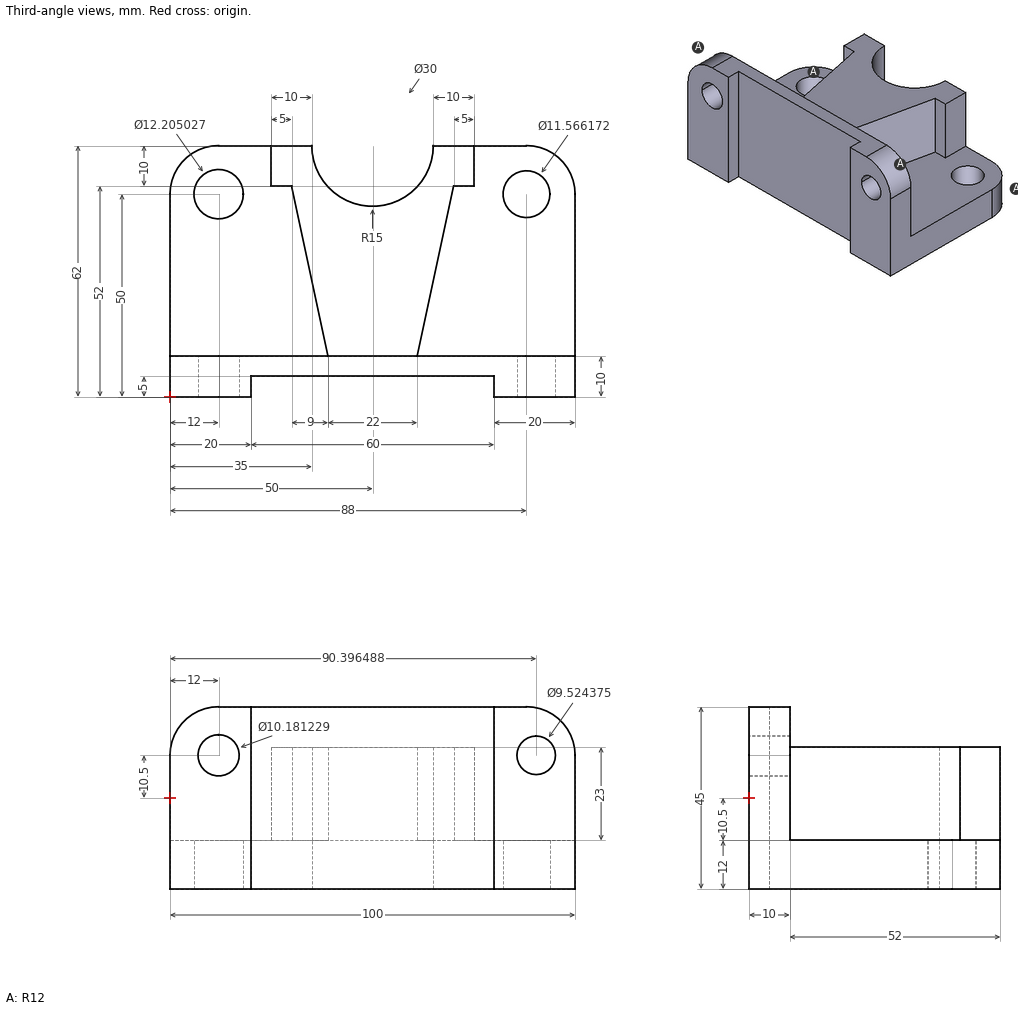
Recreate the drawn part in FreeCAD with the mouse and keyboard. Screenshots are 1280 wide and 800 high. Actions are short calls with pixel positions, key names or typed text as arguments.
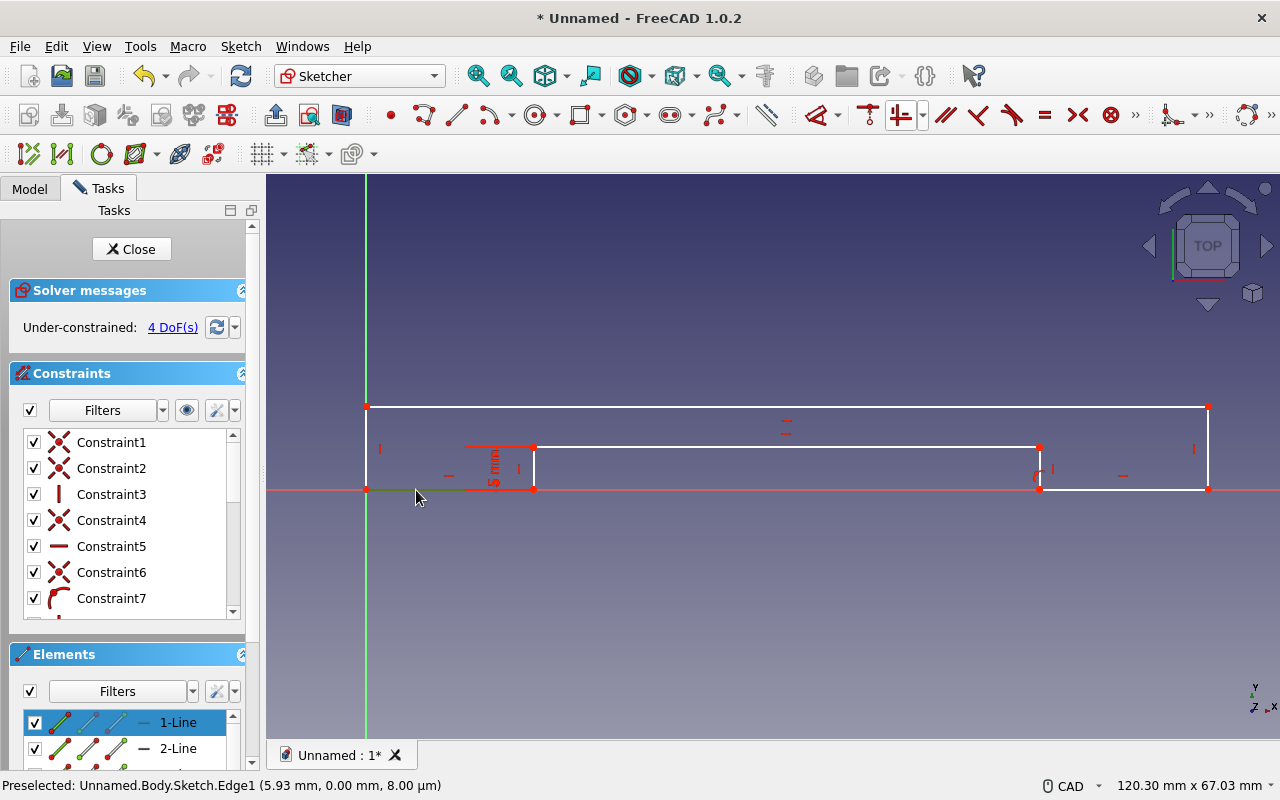
key(l)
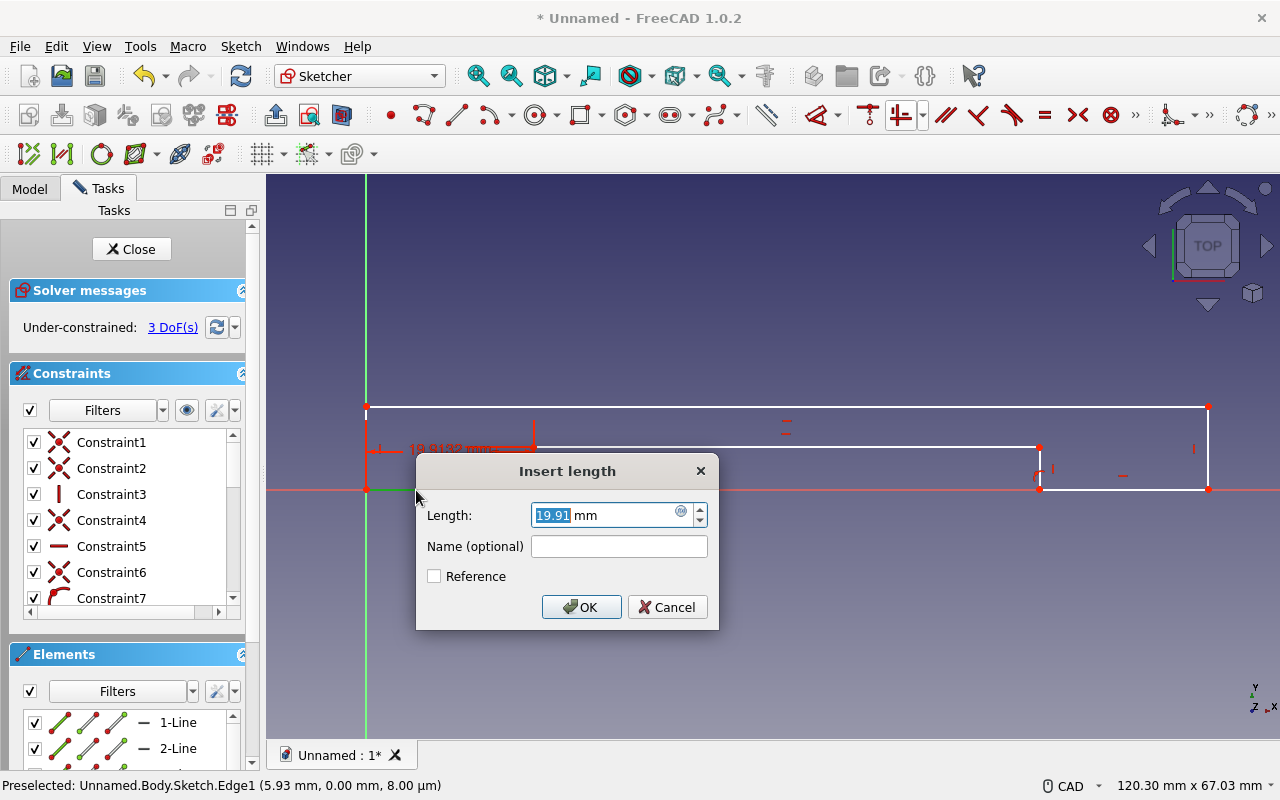
text(20)
key(Return)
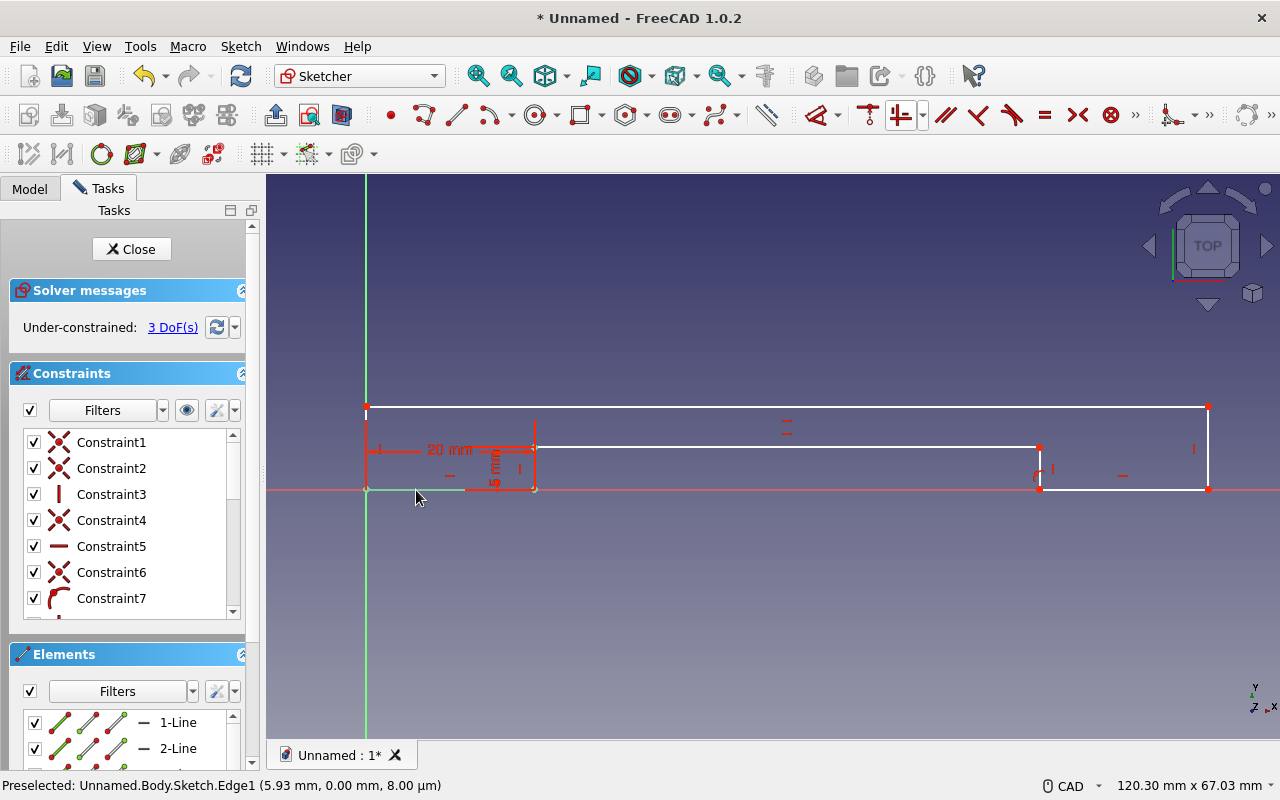
click(686, 447)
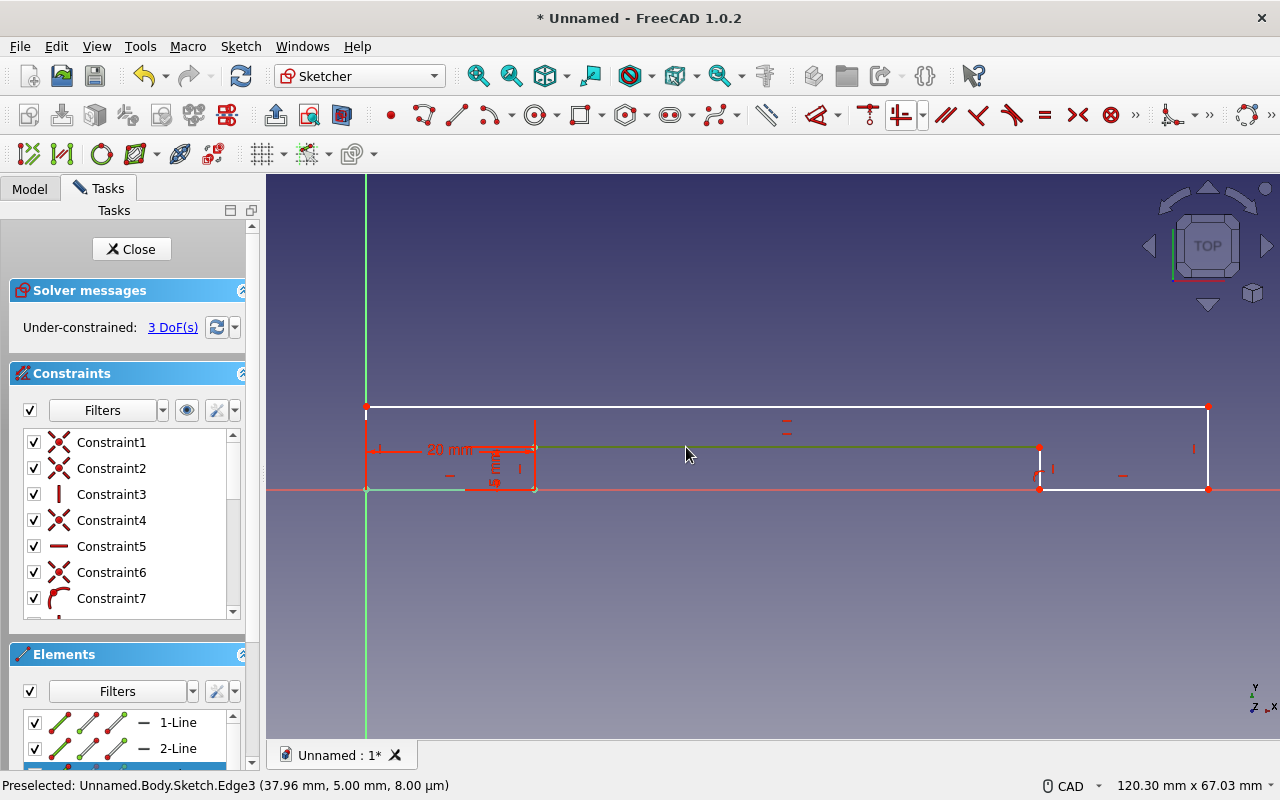
key(l)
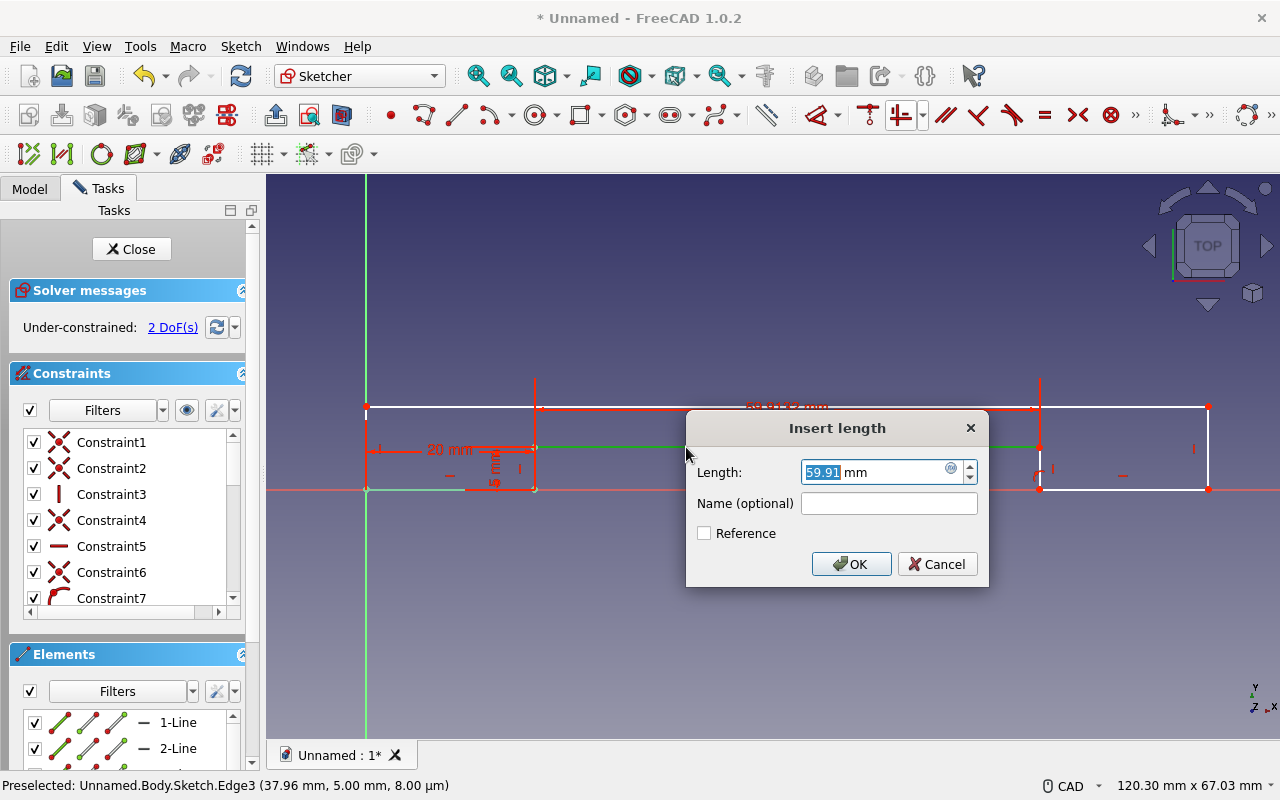
text(60)
key(Return)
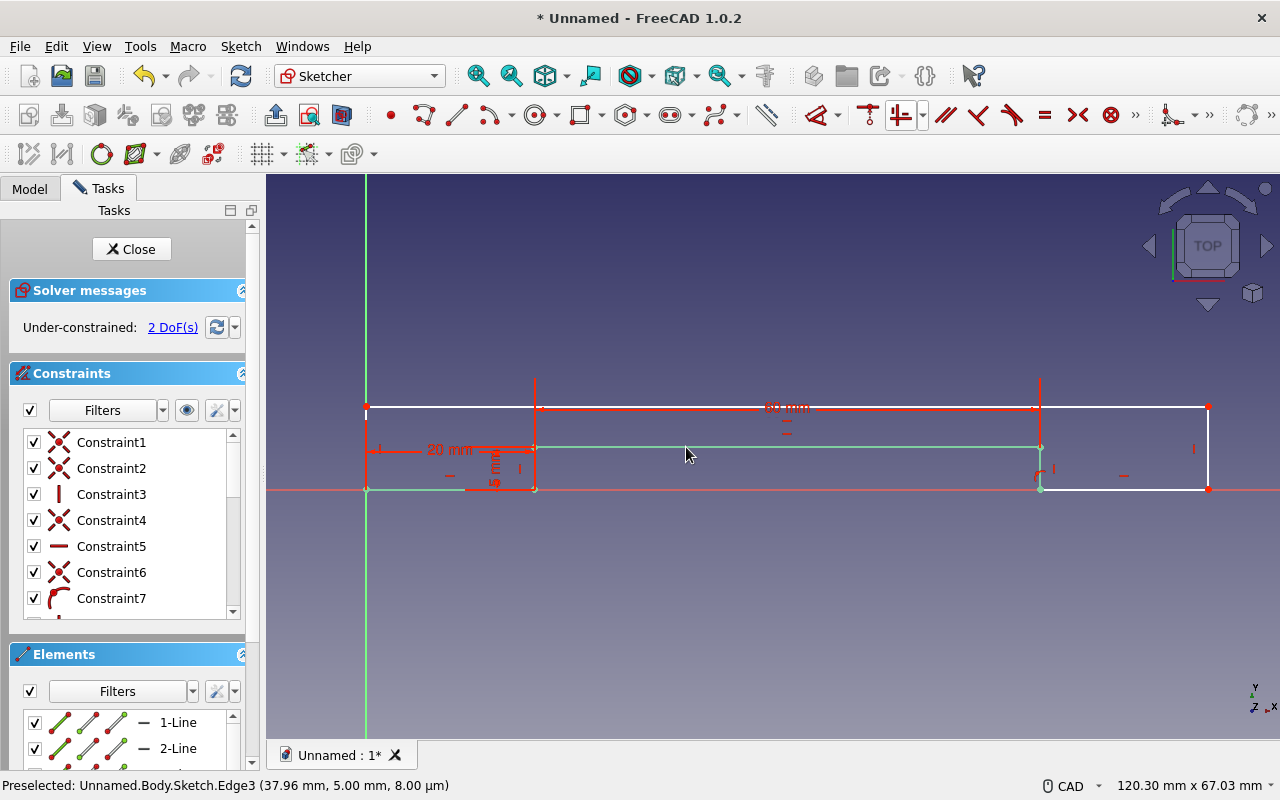
click(1091, 490)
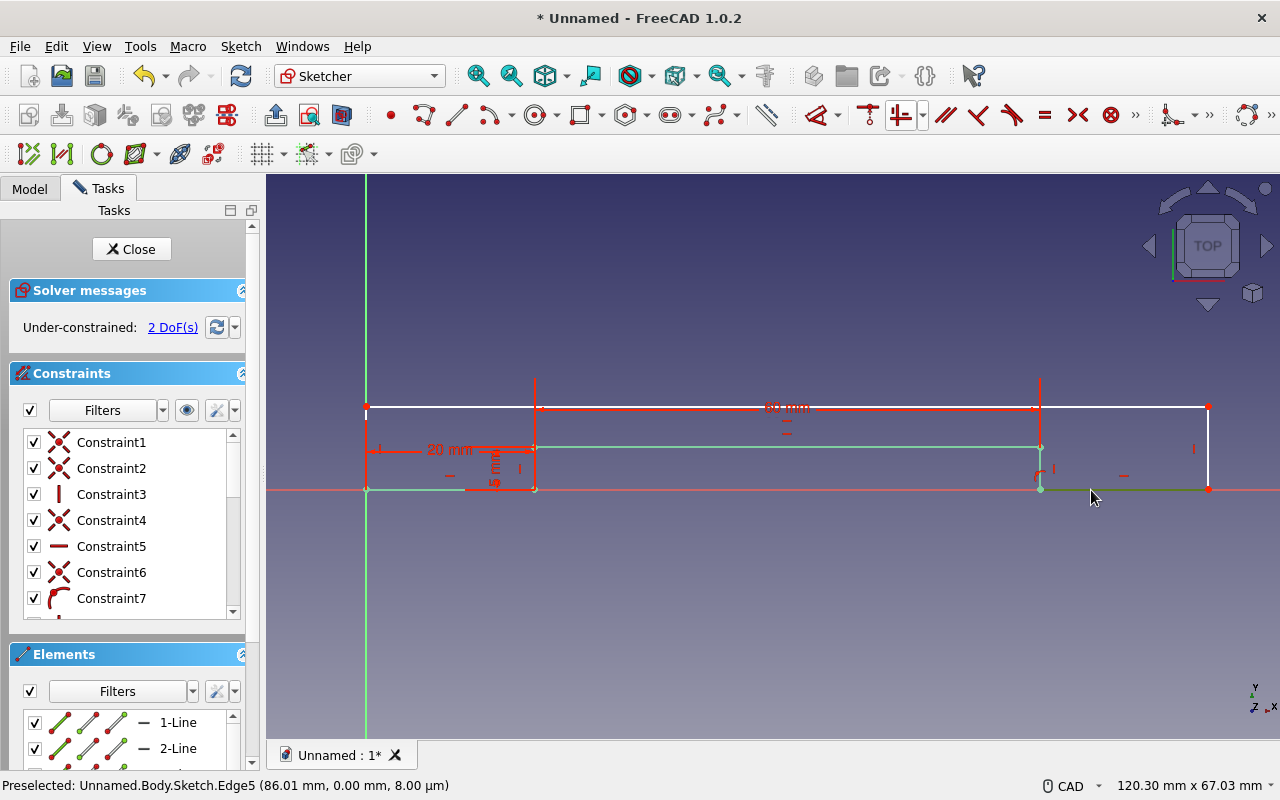
key(l)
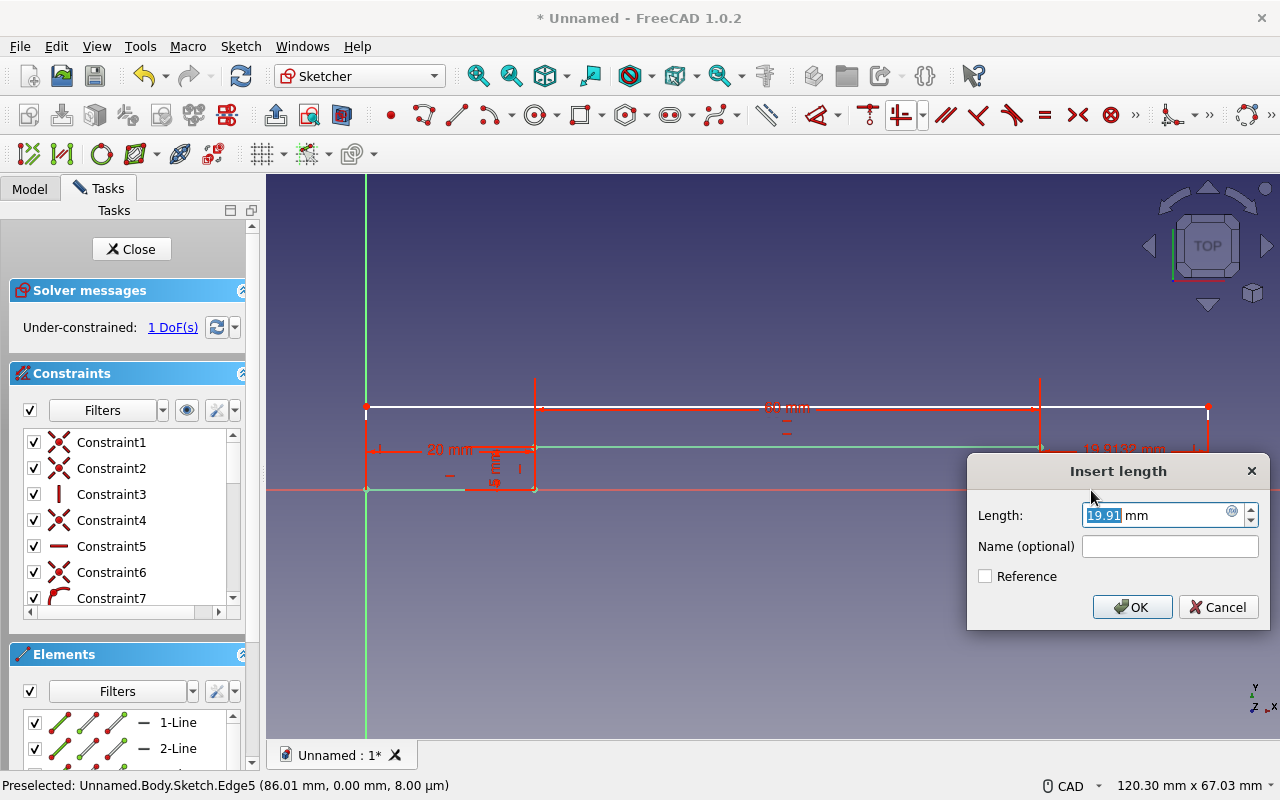
text(20)
key(Return)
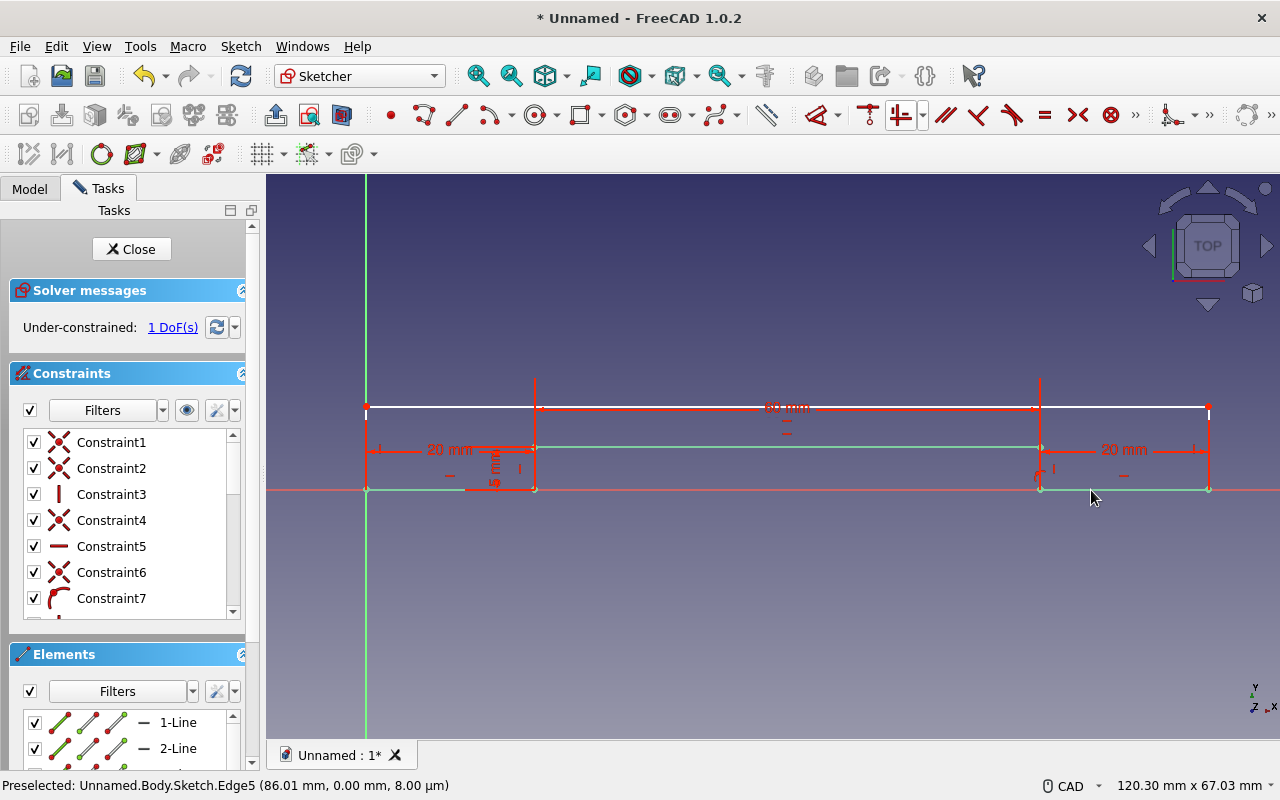
scroll(536, 475, down, 2)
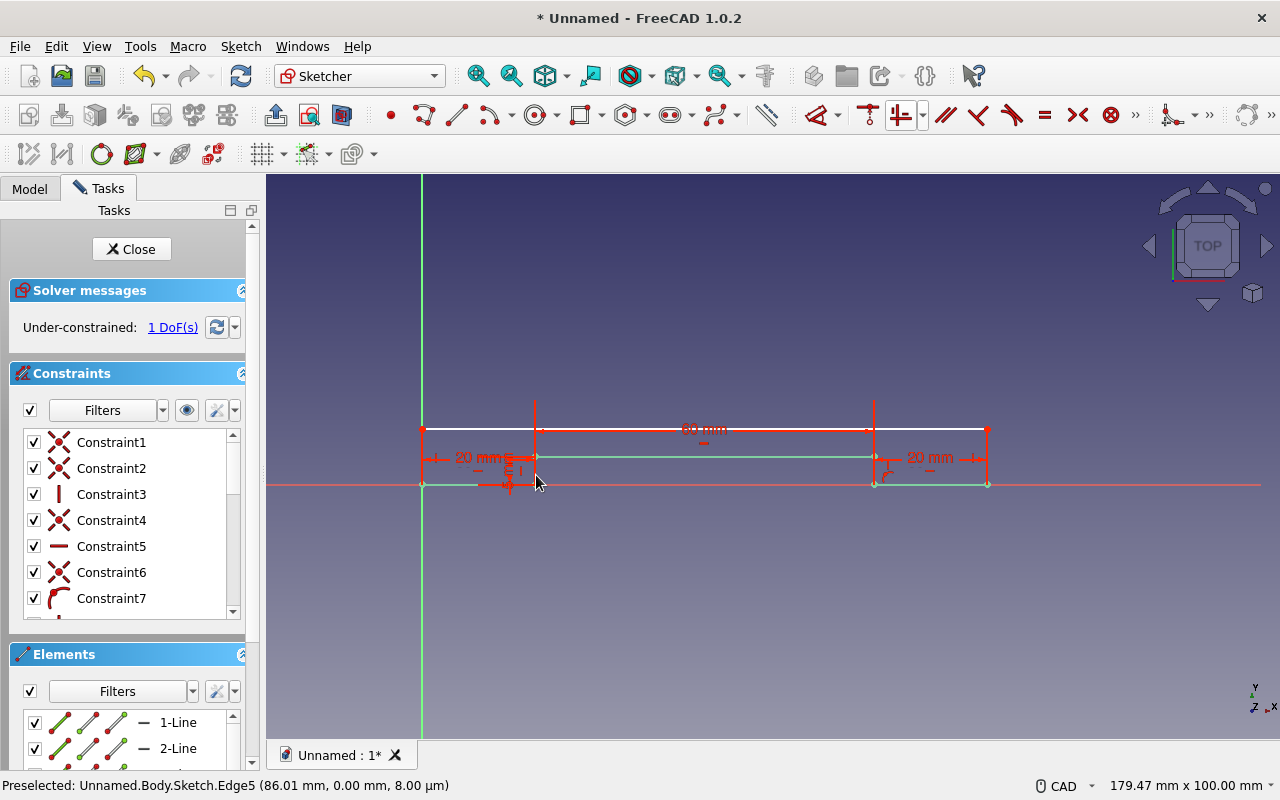
click(987, 468)